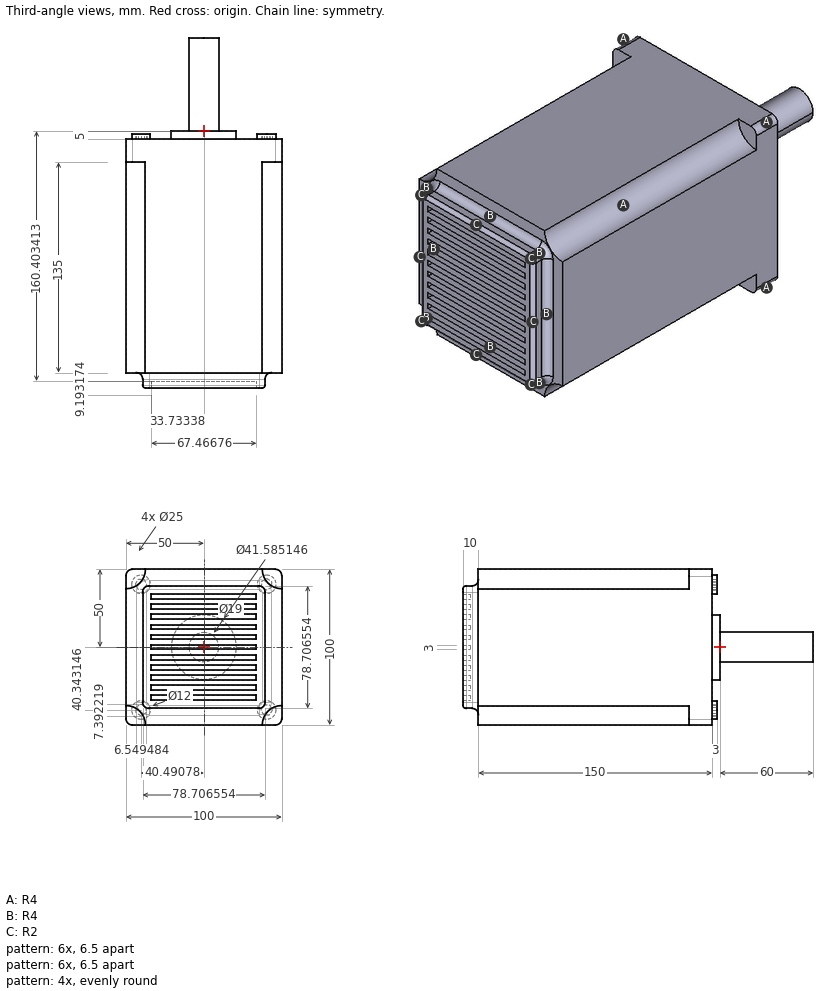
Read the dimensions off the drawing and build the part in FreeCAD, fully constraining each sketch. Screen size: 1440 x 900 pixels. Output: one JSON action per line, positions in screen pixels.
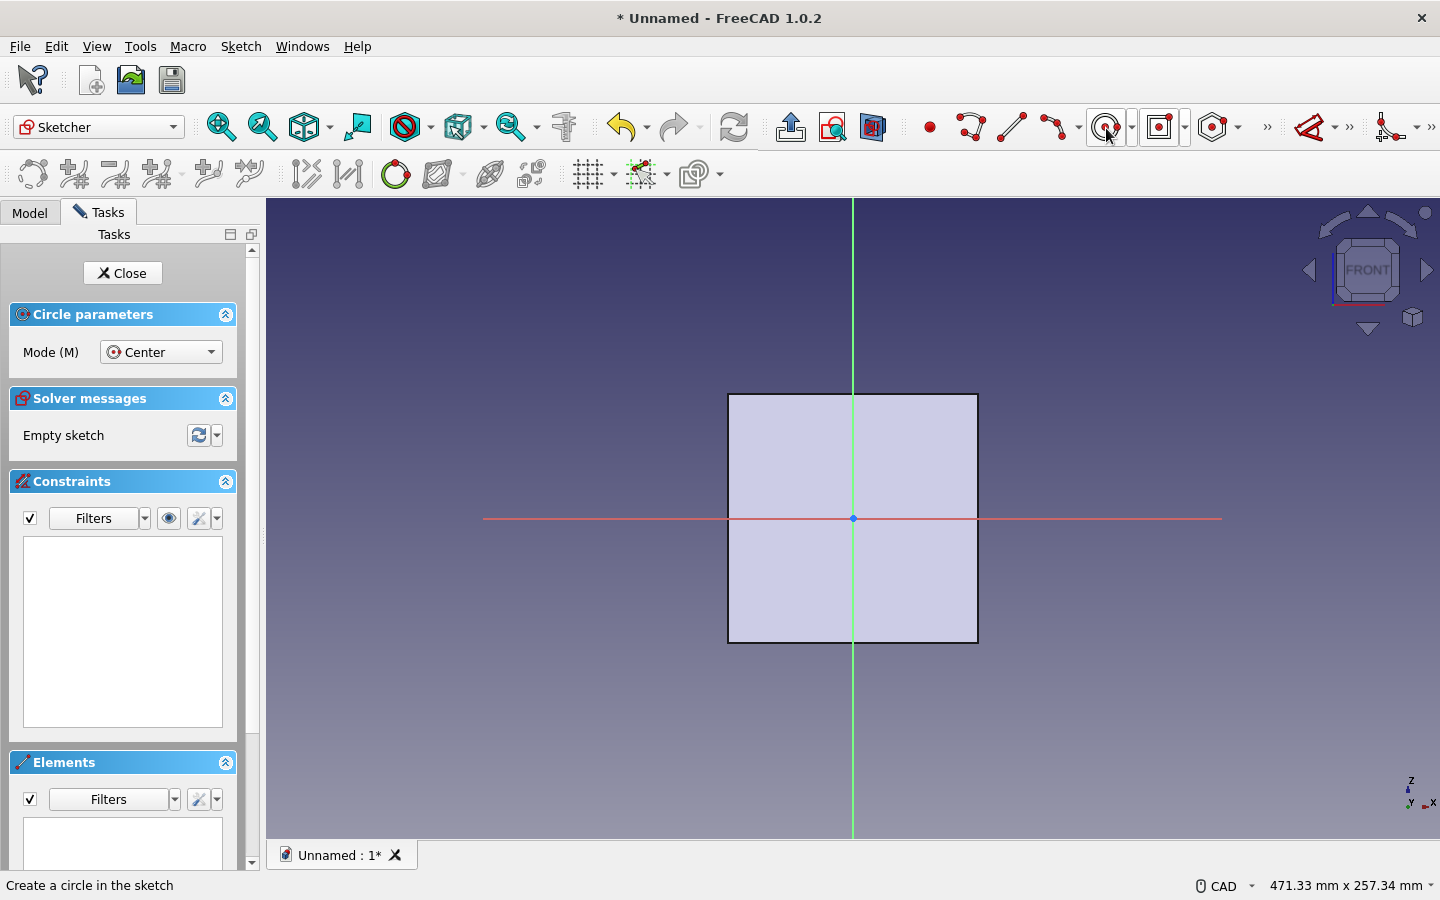
{"action": "left_click", "coordinate": [728, 394]}
{"action": "left_click", "coordinate": [750, 372]}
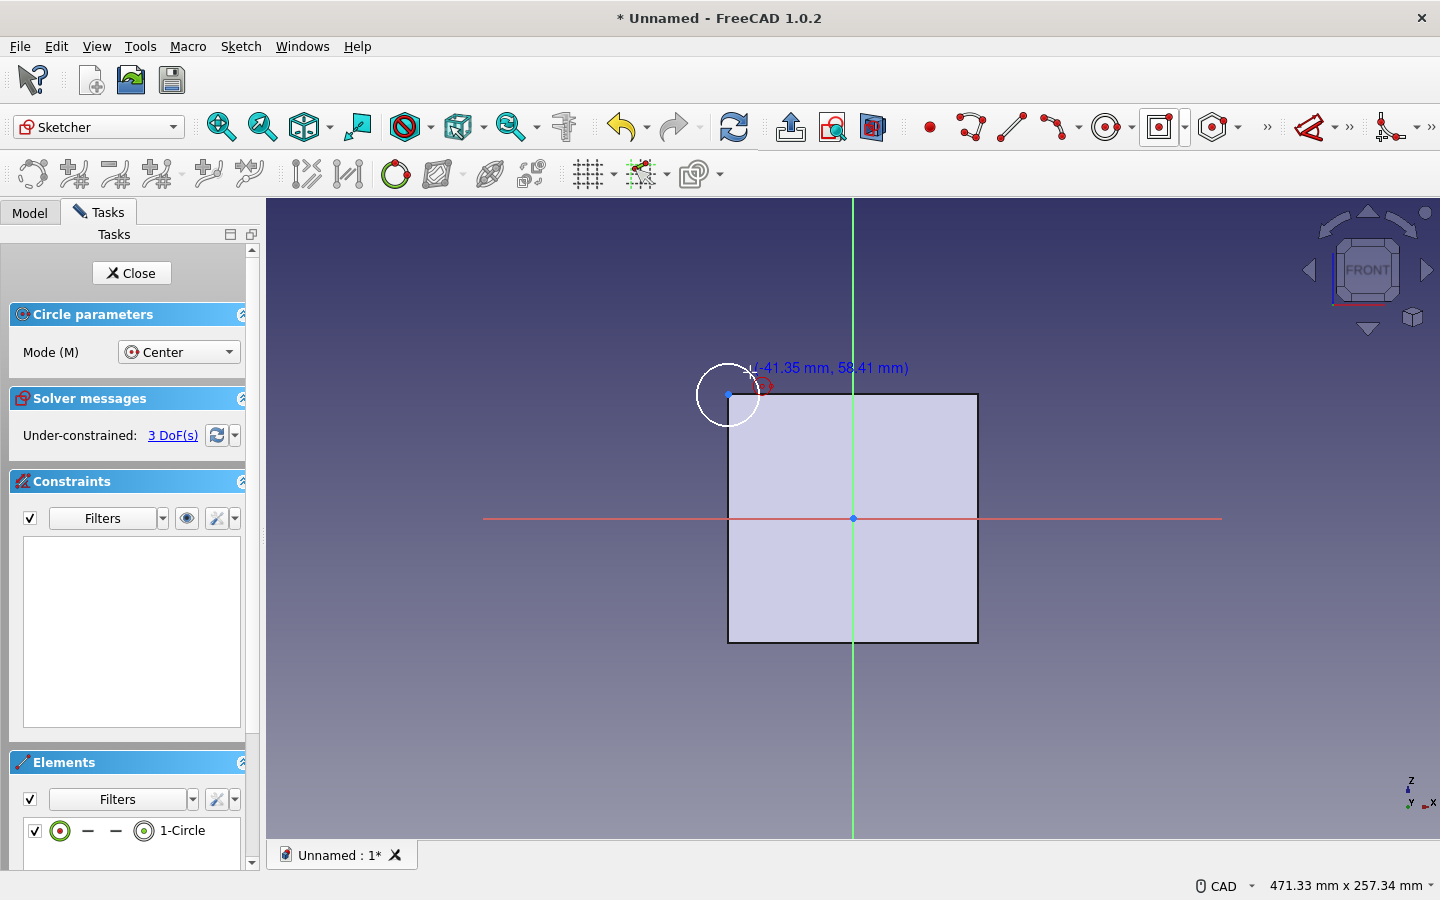
{"action": "left_click", "coordinate": [978, 394]}
{"action": "left_click", "coordinate": [1000, 372]}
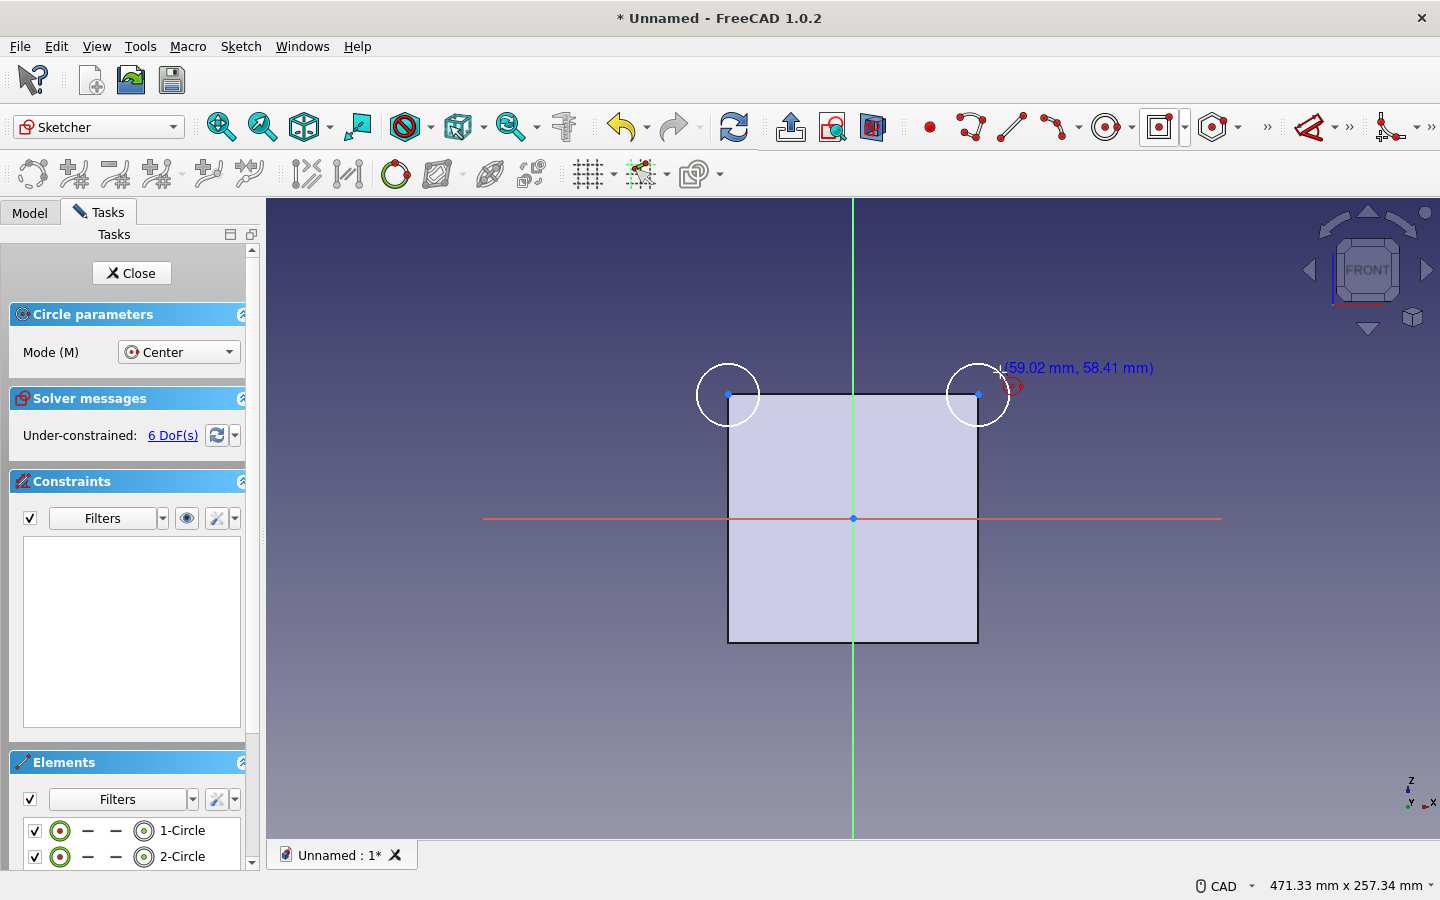
{"action": "left_click", "coordinate": [728, 643]}
{"action": "left_click", "coordinate": [750, 621]}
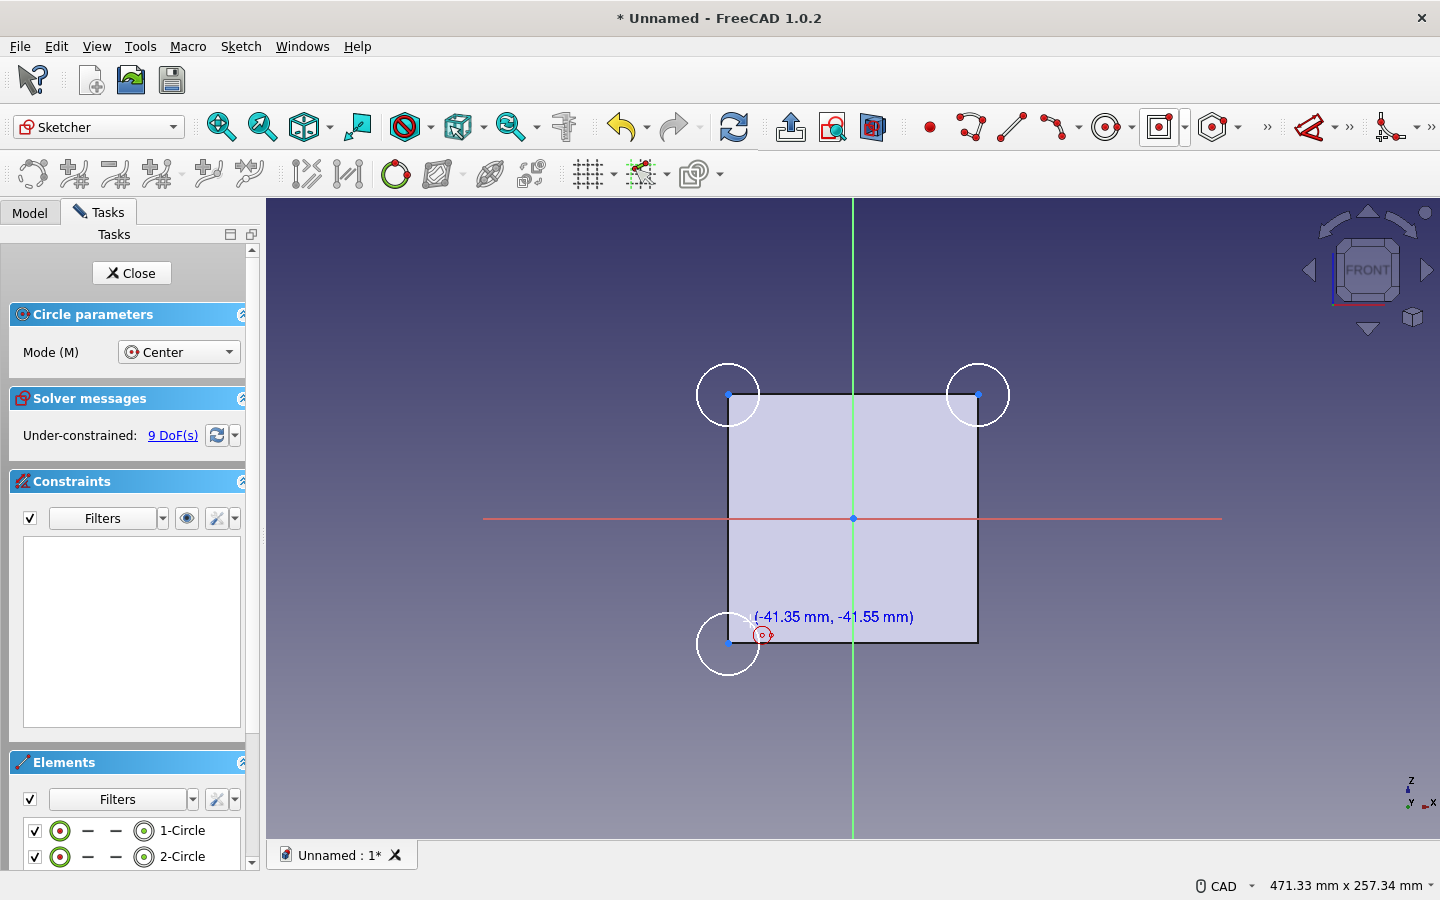
{"action": "left_click", "coordinate": [978, 643]}
{"action": "left_click", "coordinate": [1000, 621]}
{"action": "key", "text": "Escape"}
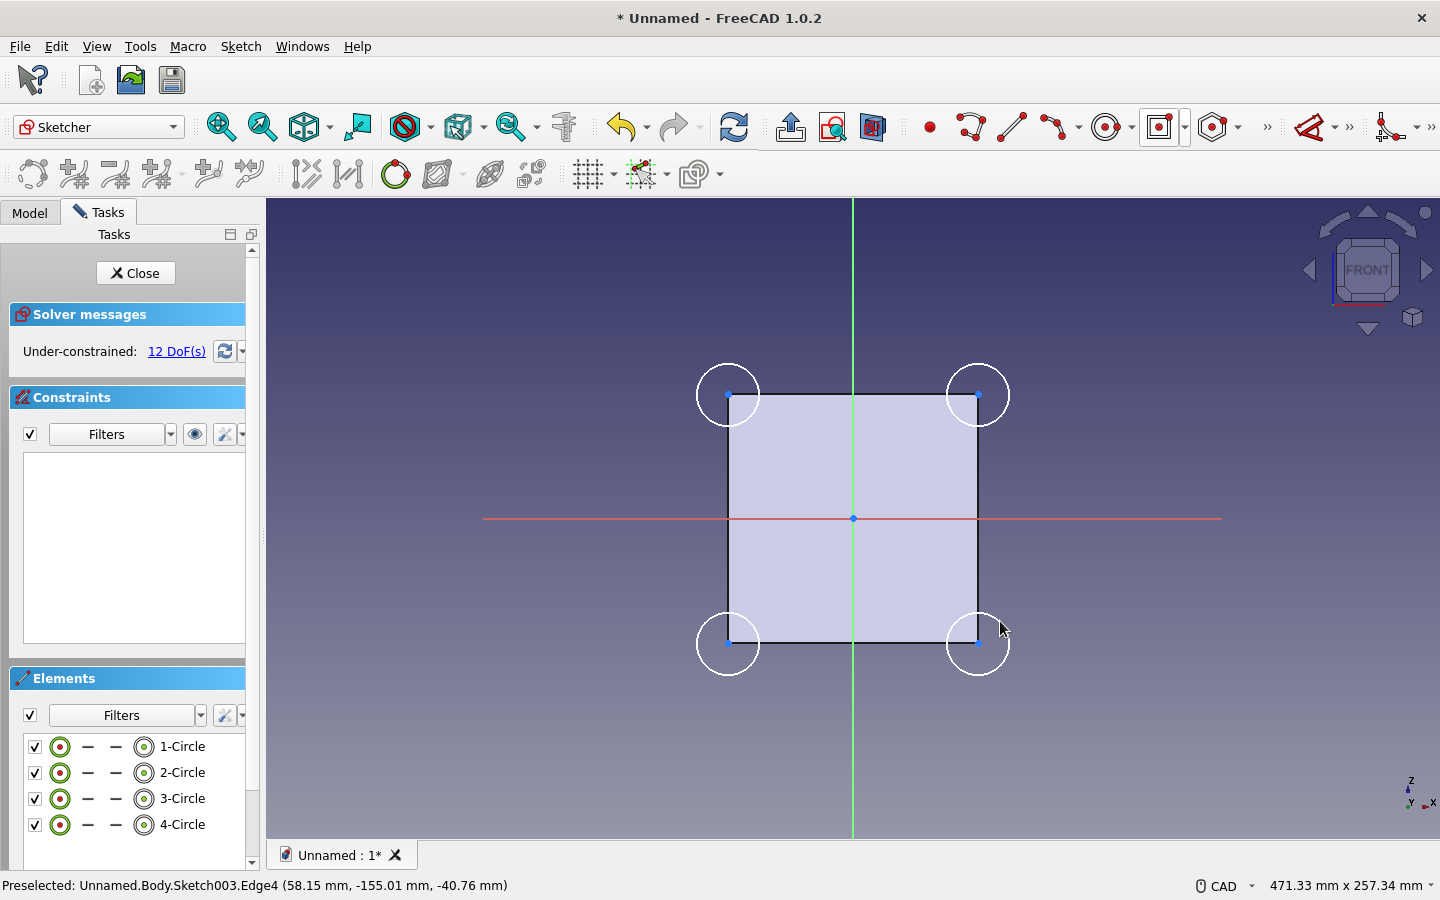
{"action": "left_click", "coordinate": [750, 373]}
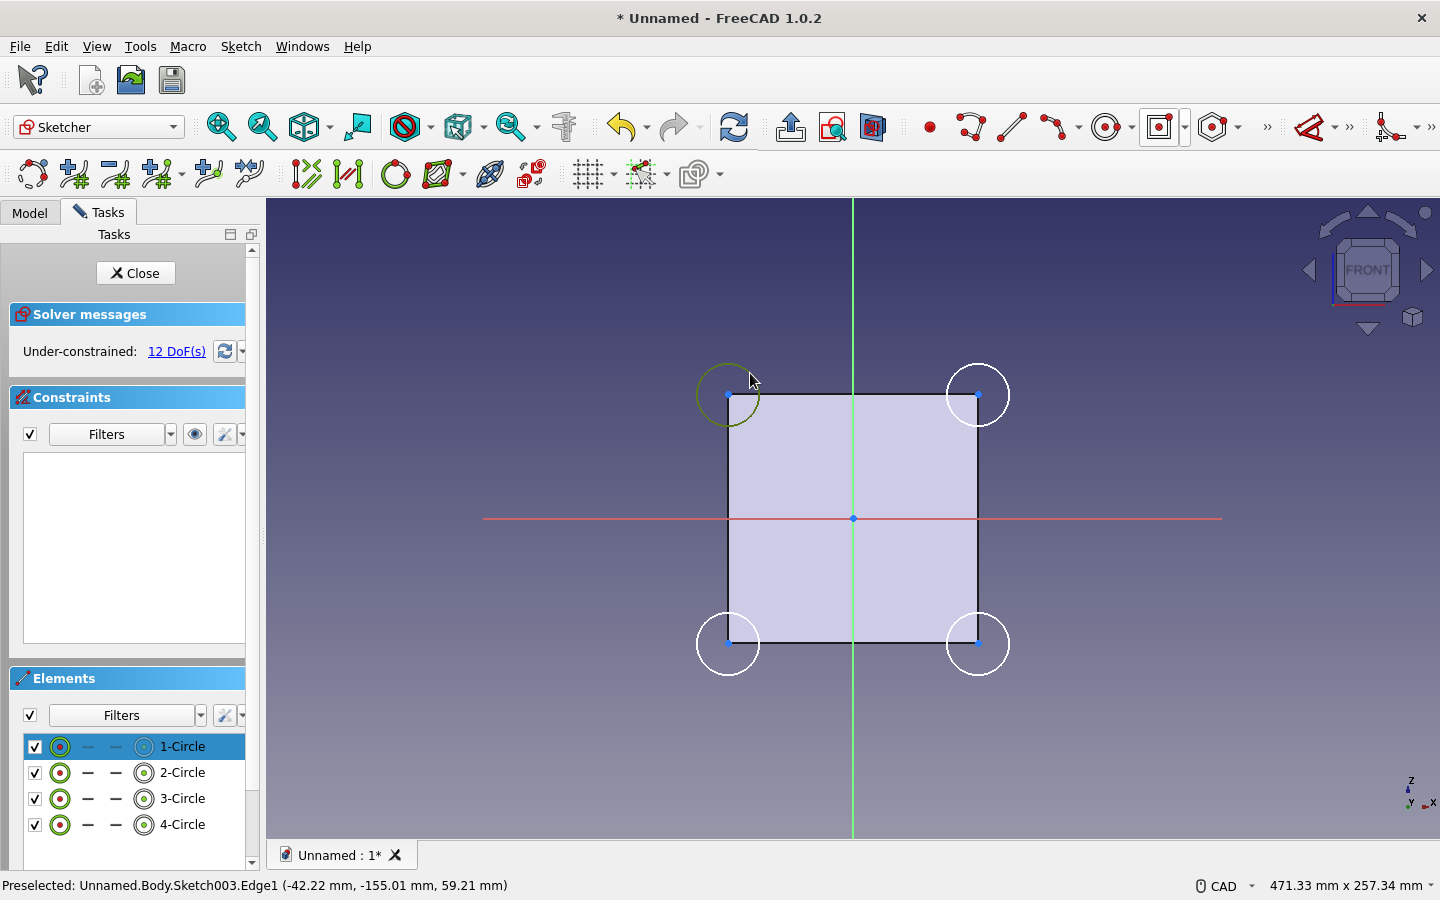
{"action": "left_click", "coordinate": [1000, 373]}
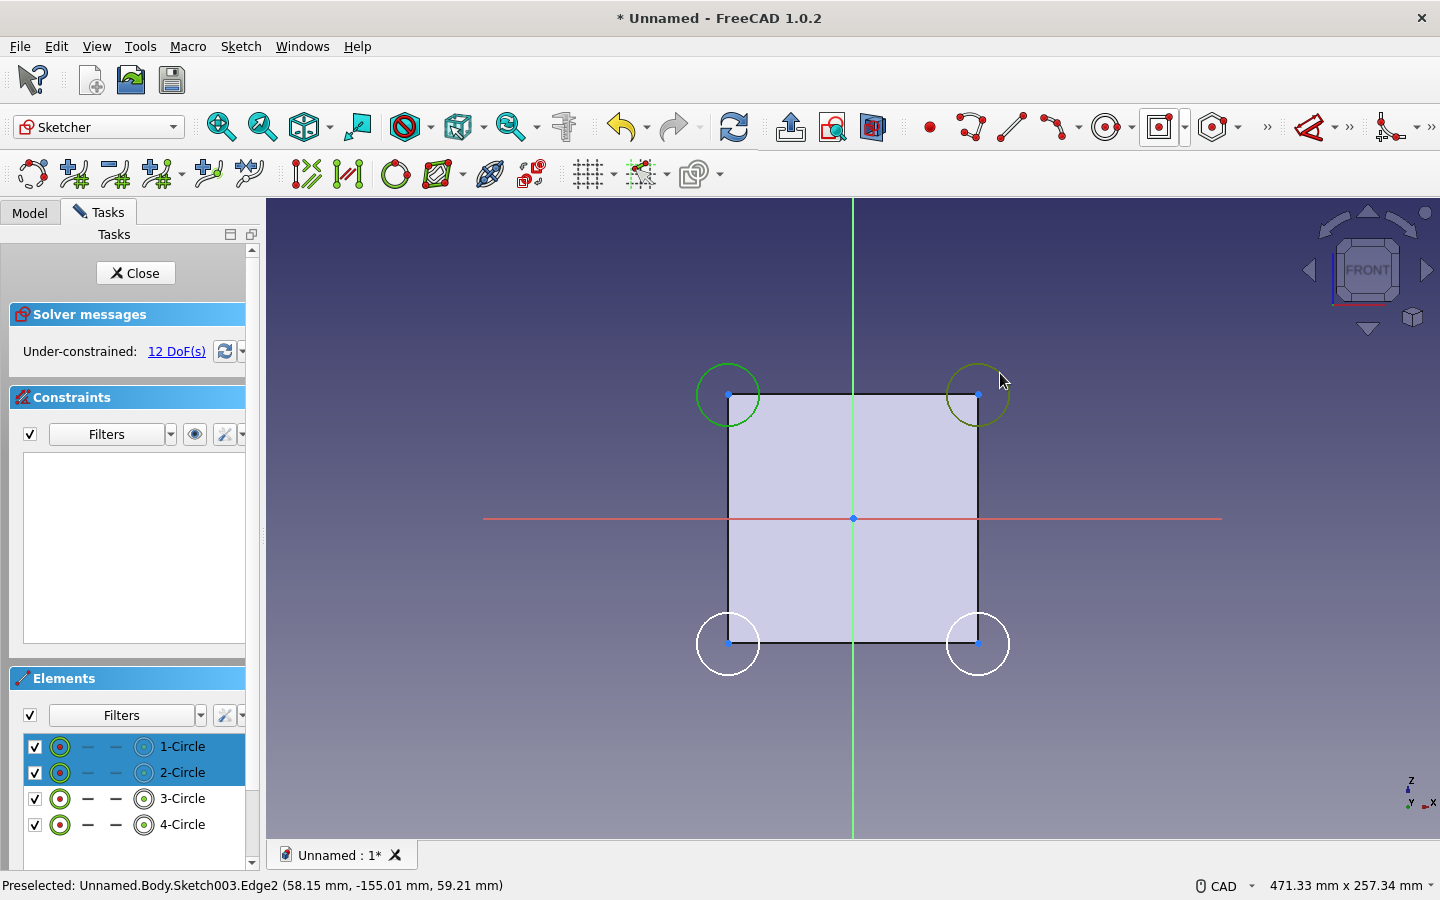
{"action": "left_click", "coordinate": [750, 622]}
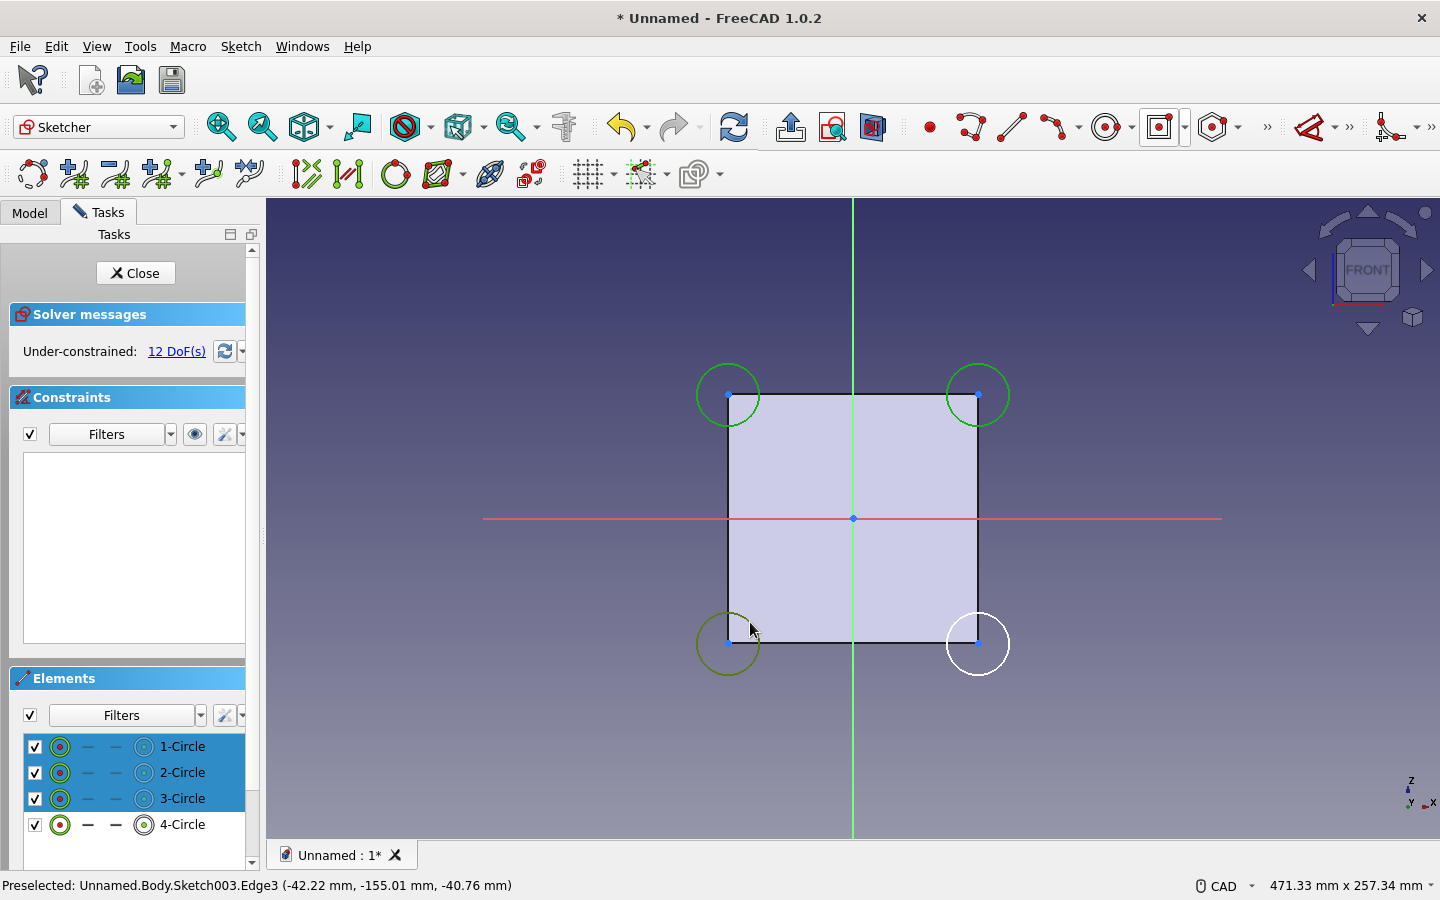
{"action": "left_click", "coordinate": [1000, 622]}